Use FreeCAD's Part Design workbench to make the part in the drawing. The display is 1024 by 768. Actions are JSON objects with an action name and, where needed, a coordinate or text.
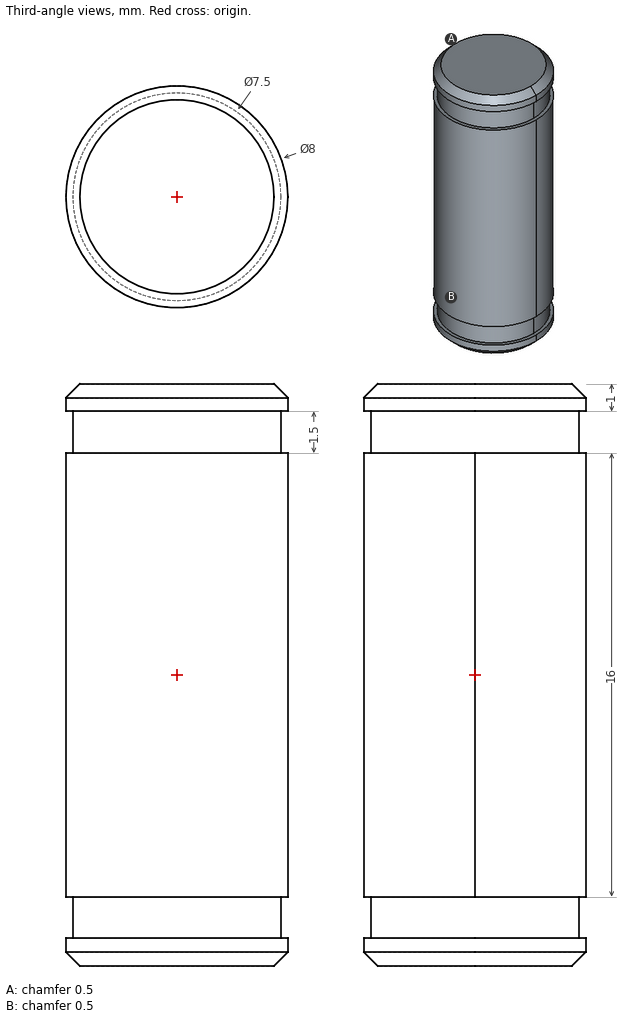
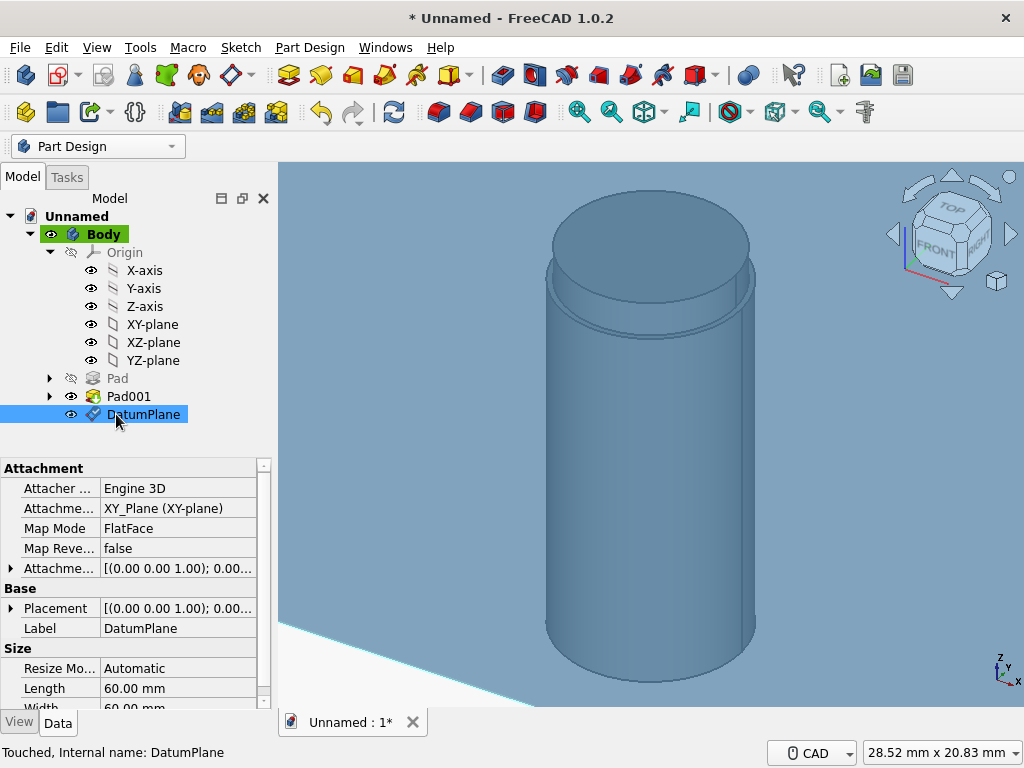
{"action": "left_click", "coordinate": [58, 76]}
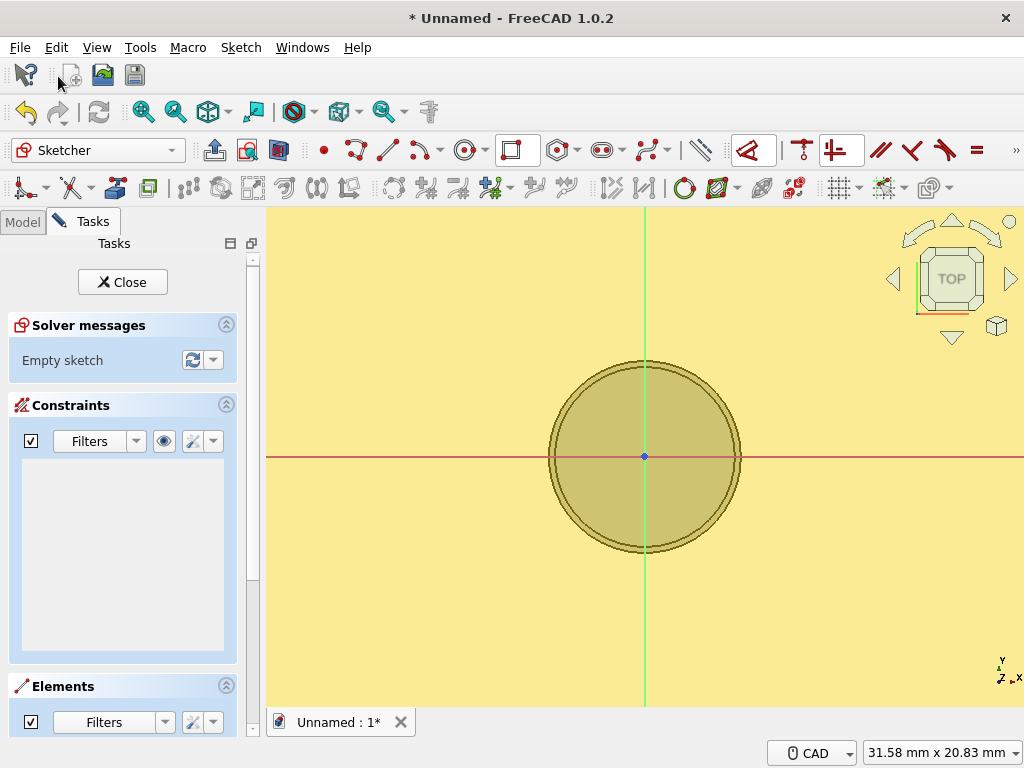
{"action": "scroll", "coordinate": [784, 457], "scroll_direction": "up", "scroll_amount": 2}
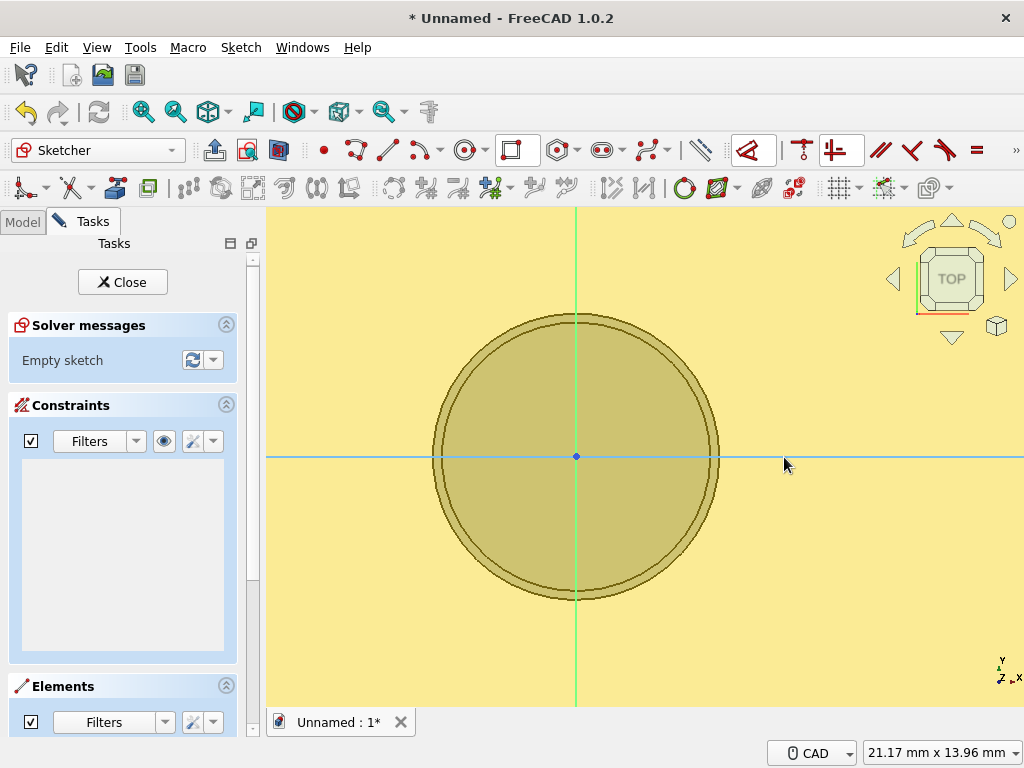
{"action": "key", "text": "g c"}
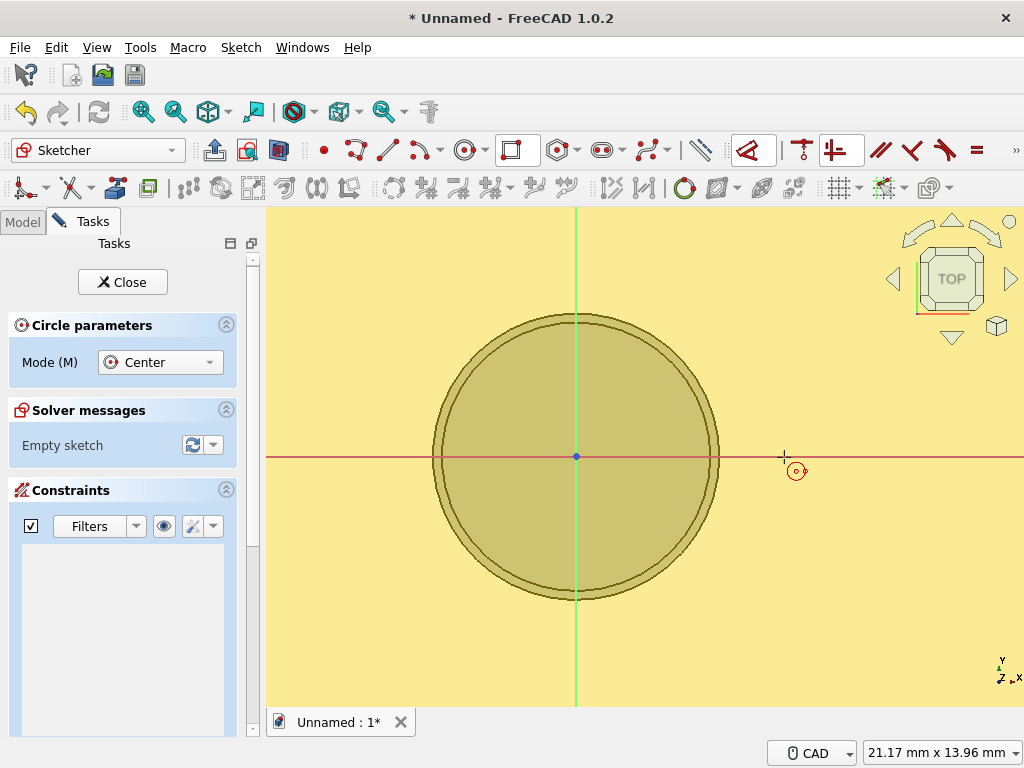
{"action": "left_click", "coordinate": [576, 457]}
{"action": "left_click", "coordinate": [677, 355]}
{"action": "key", "text": "Escape"}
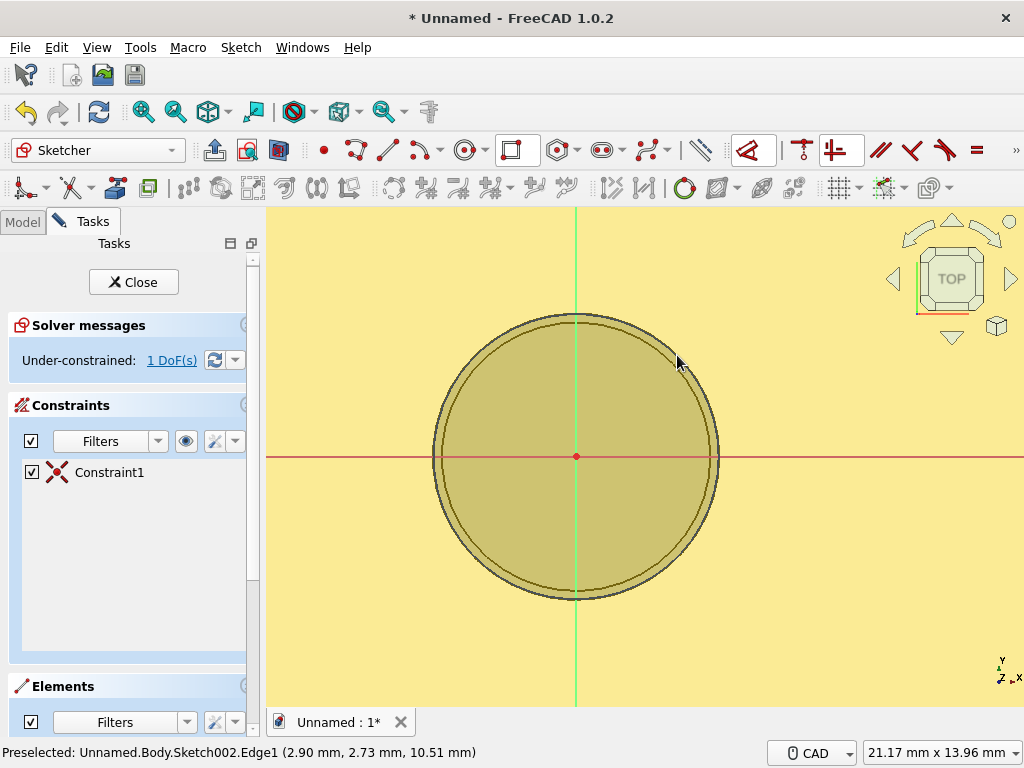
{"action": "left_click", "coordinate": [677, 356]}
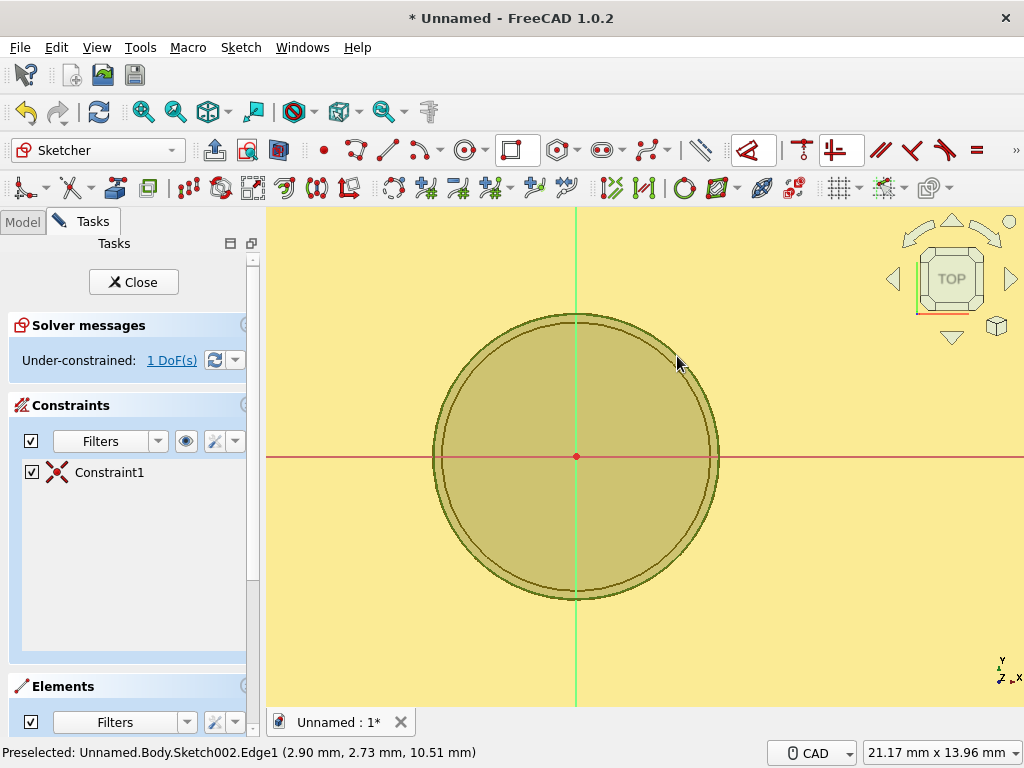
{"action": "key", "text": "k o"}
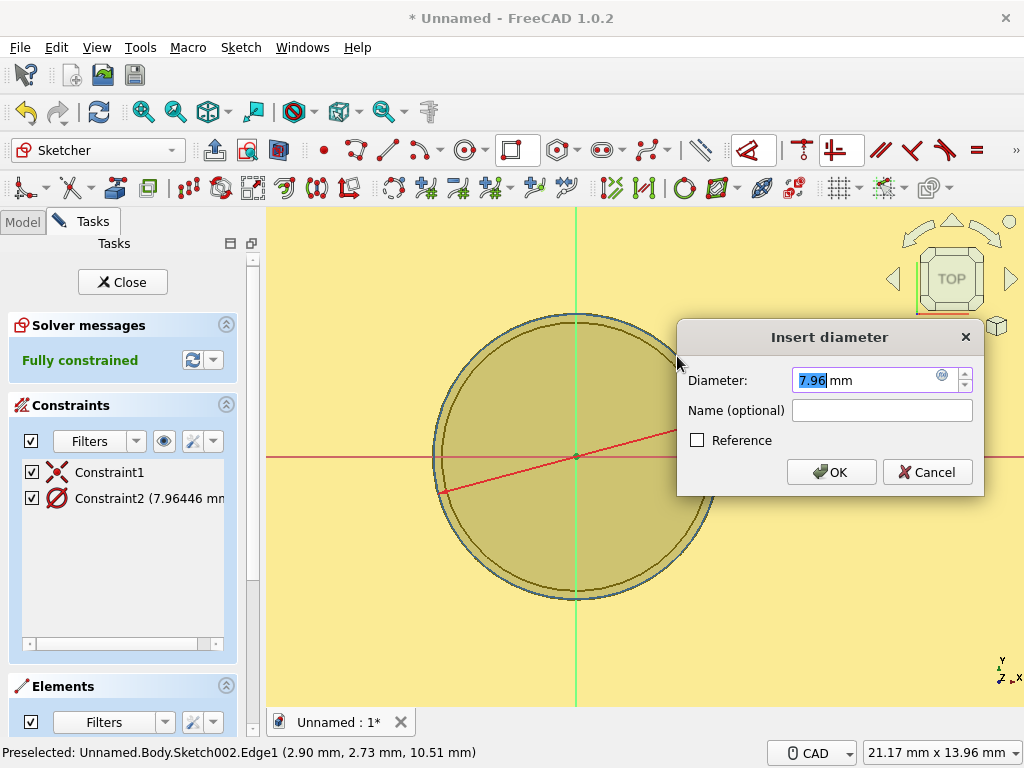
{"action": "type", "text": "8"}
{"action": "key", "text": "Return"}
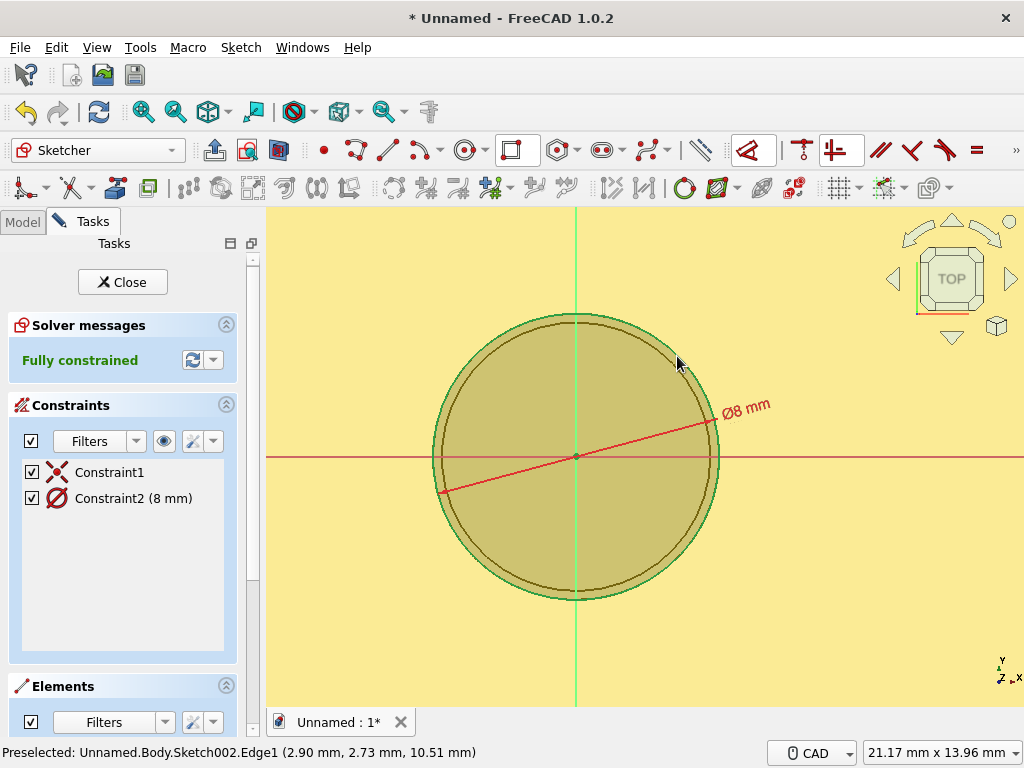
{"action": "left_click", "coordinate": [123, 282]}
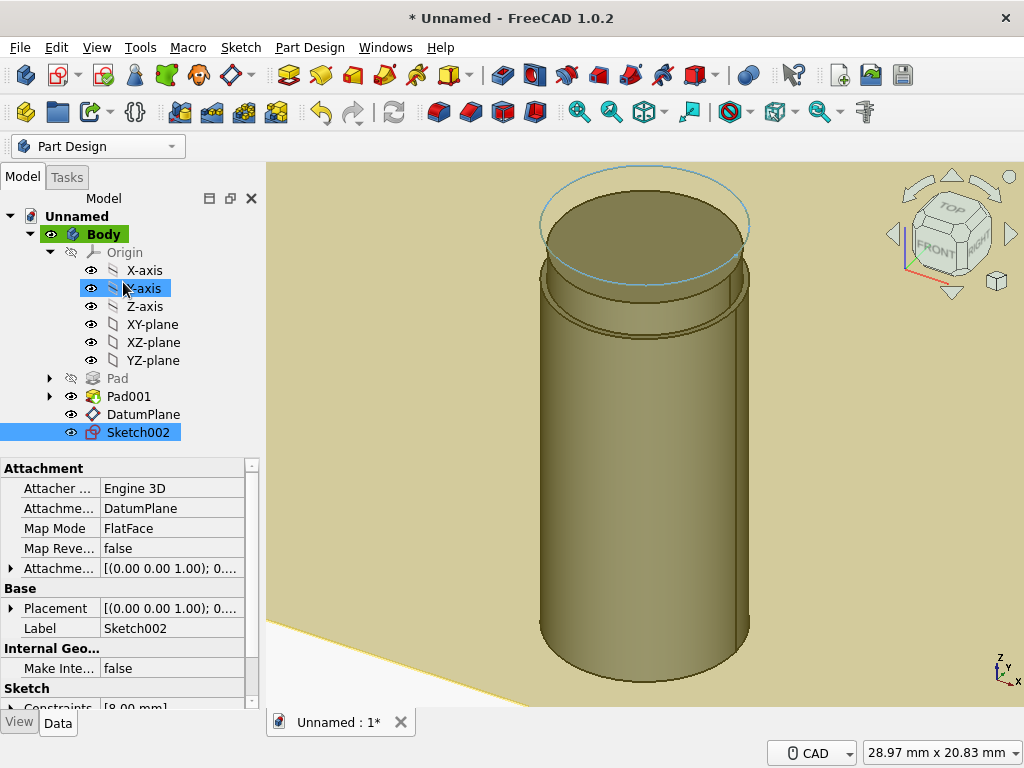
{"action": "left_click", "coordinate": [290, 76]}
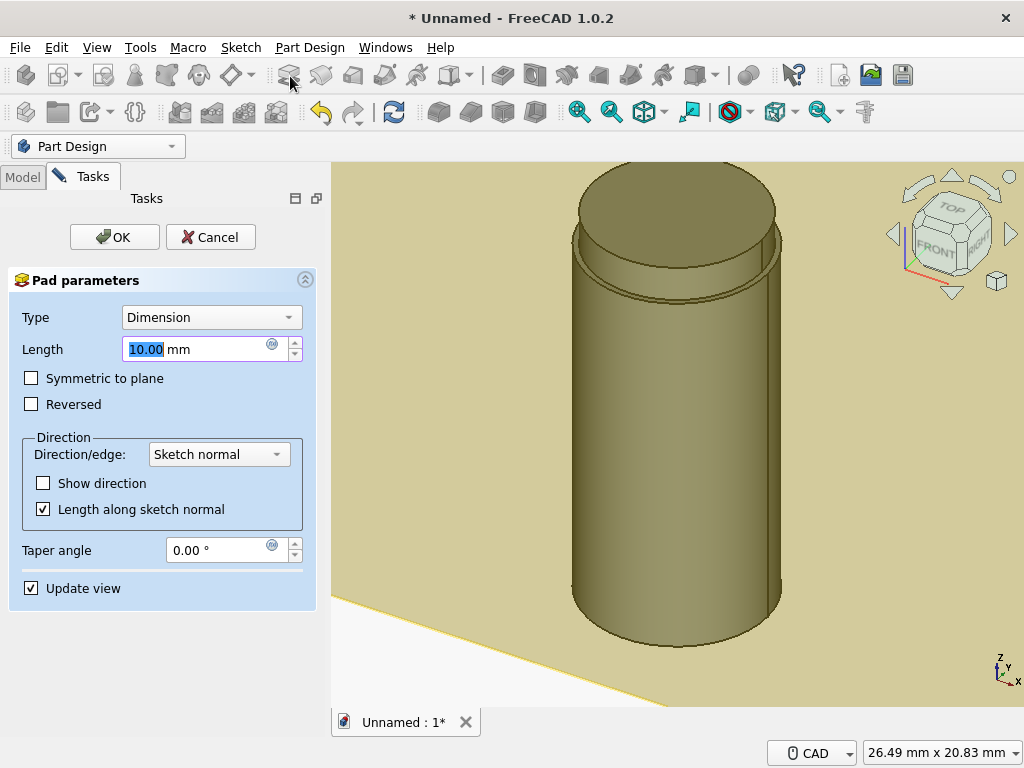
{"action": "type", "text": "1"}
{"action": "key", "text": "Tab"}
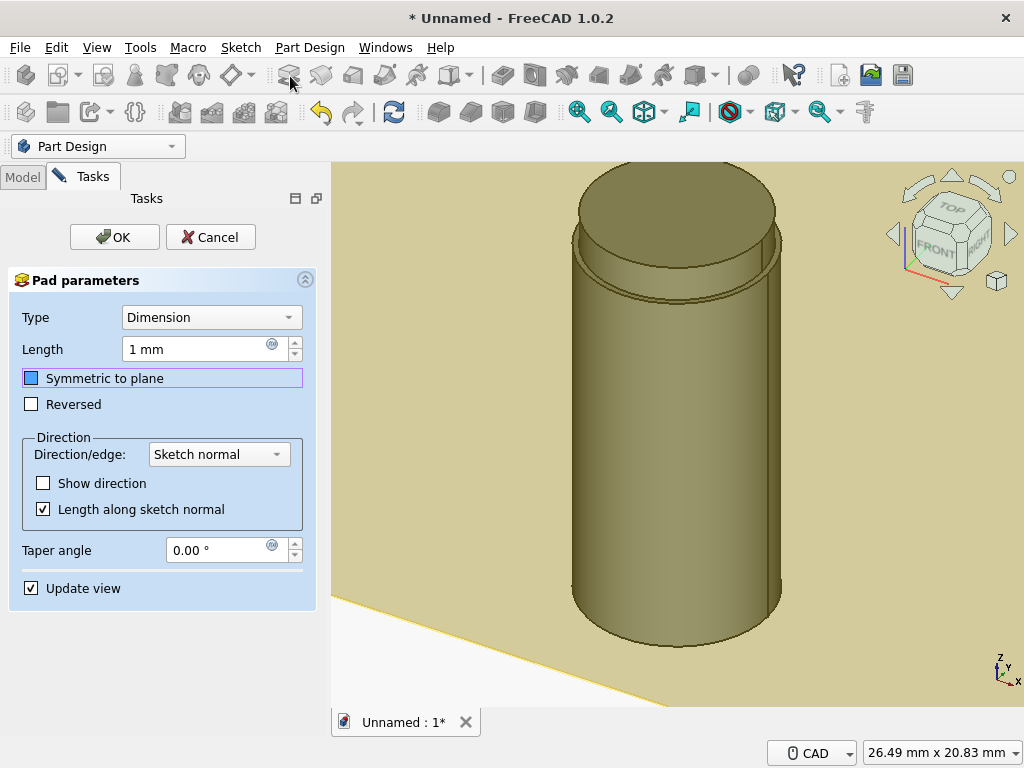
{"action": "left_click", "coordinate": [30, 404]}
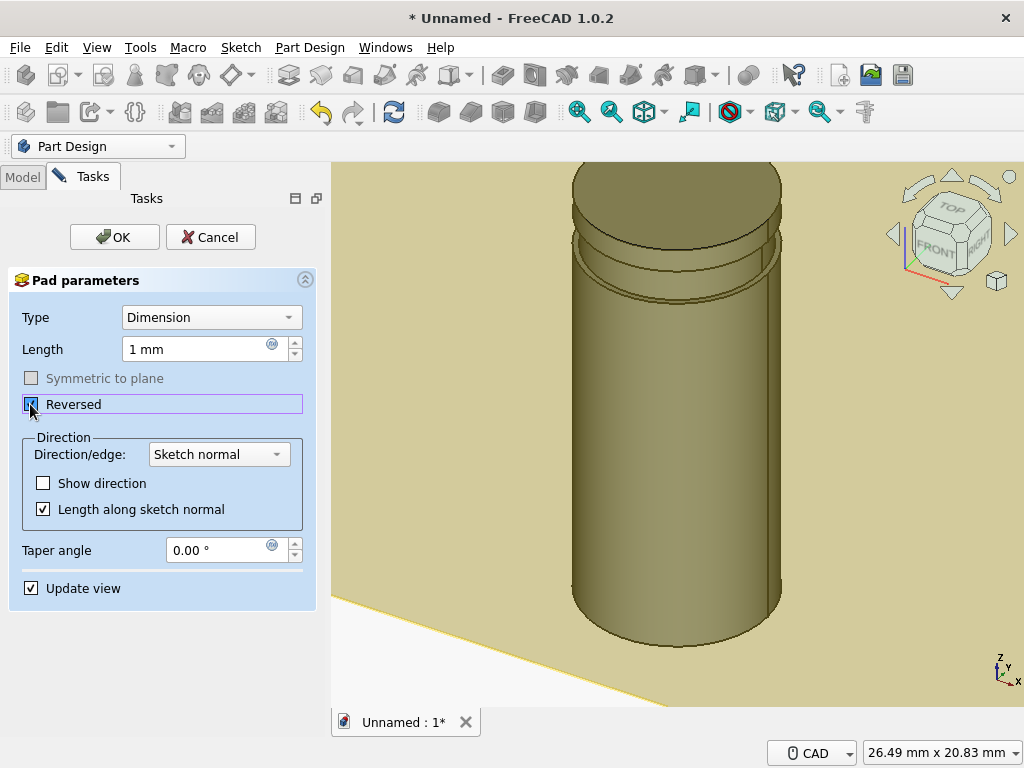
{"action": "left_click", "coordinate": [115, 237]}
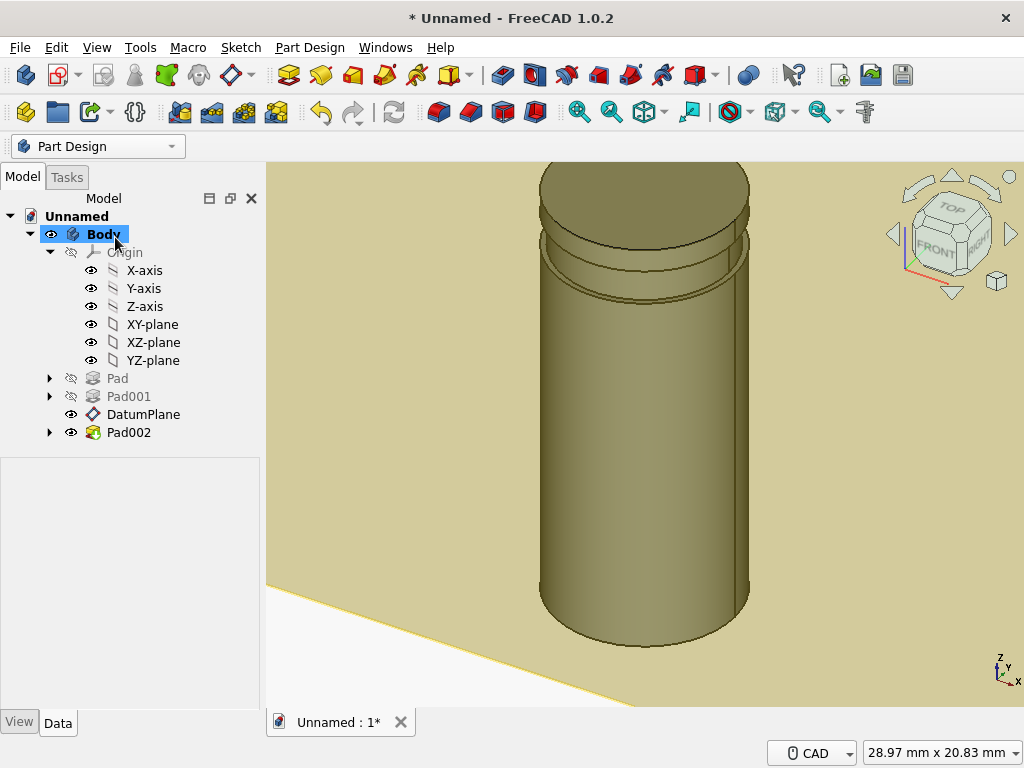
{"action": "left_click", "coordinate": [116, 414]}
{"action": "key", "text": "space"}